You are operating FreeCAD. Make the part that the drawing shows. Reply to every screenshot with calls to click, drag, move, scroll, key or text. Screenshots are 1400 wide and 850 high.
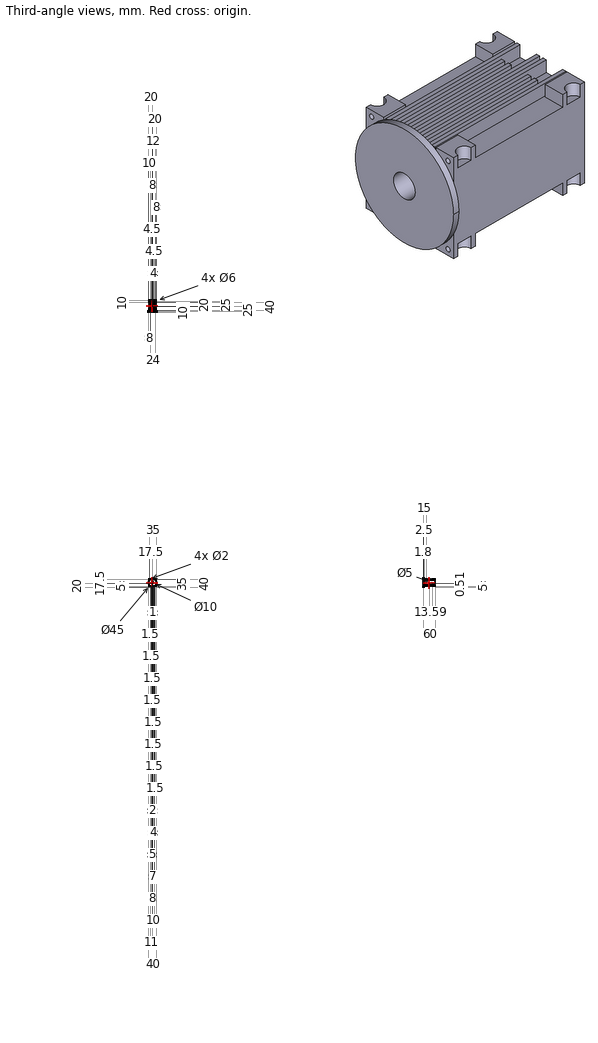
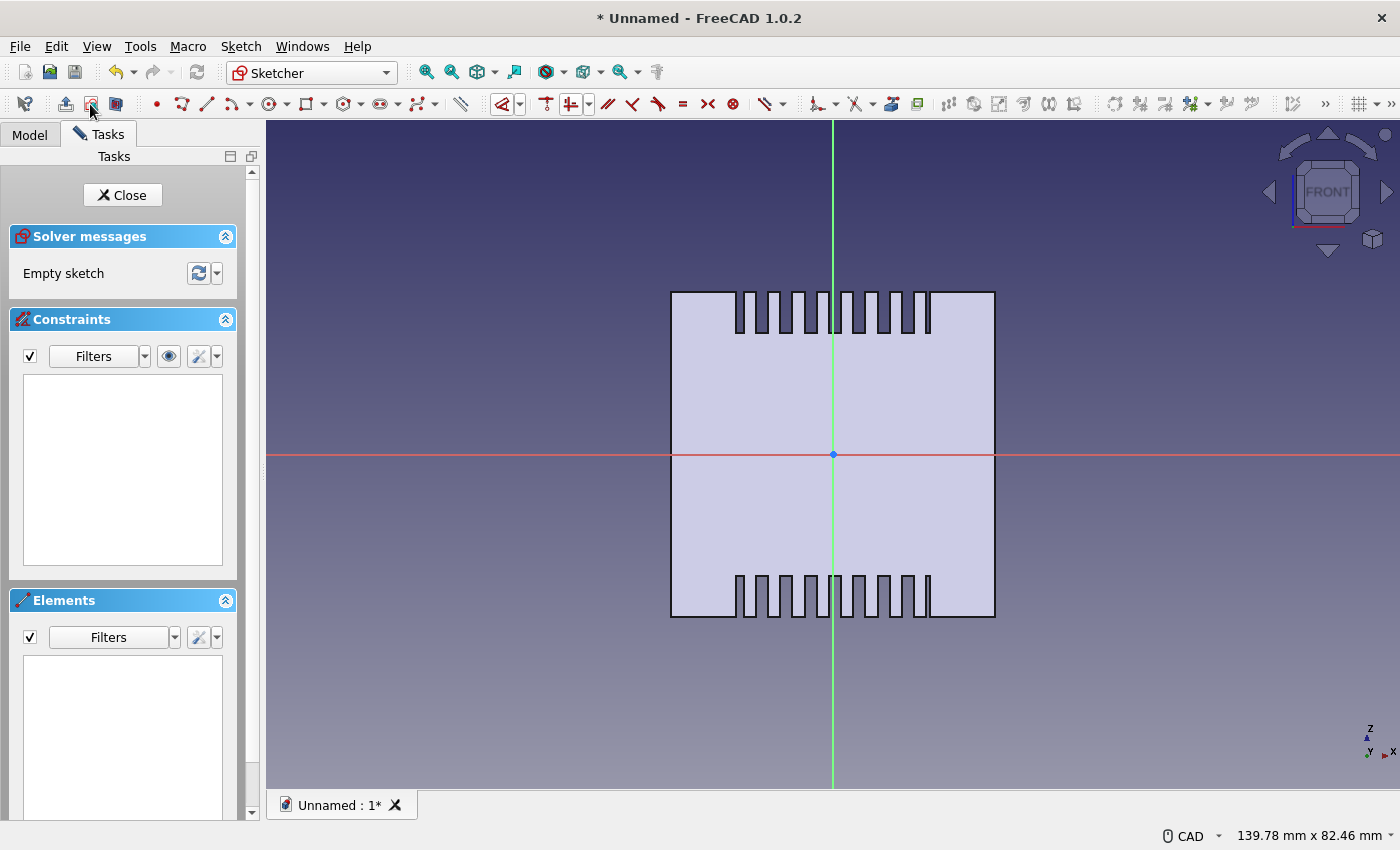
click(268, 104)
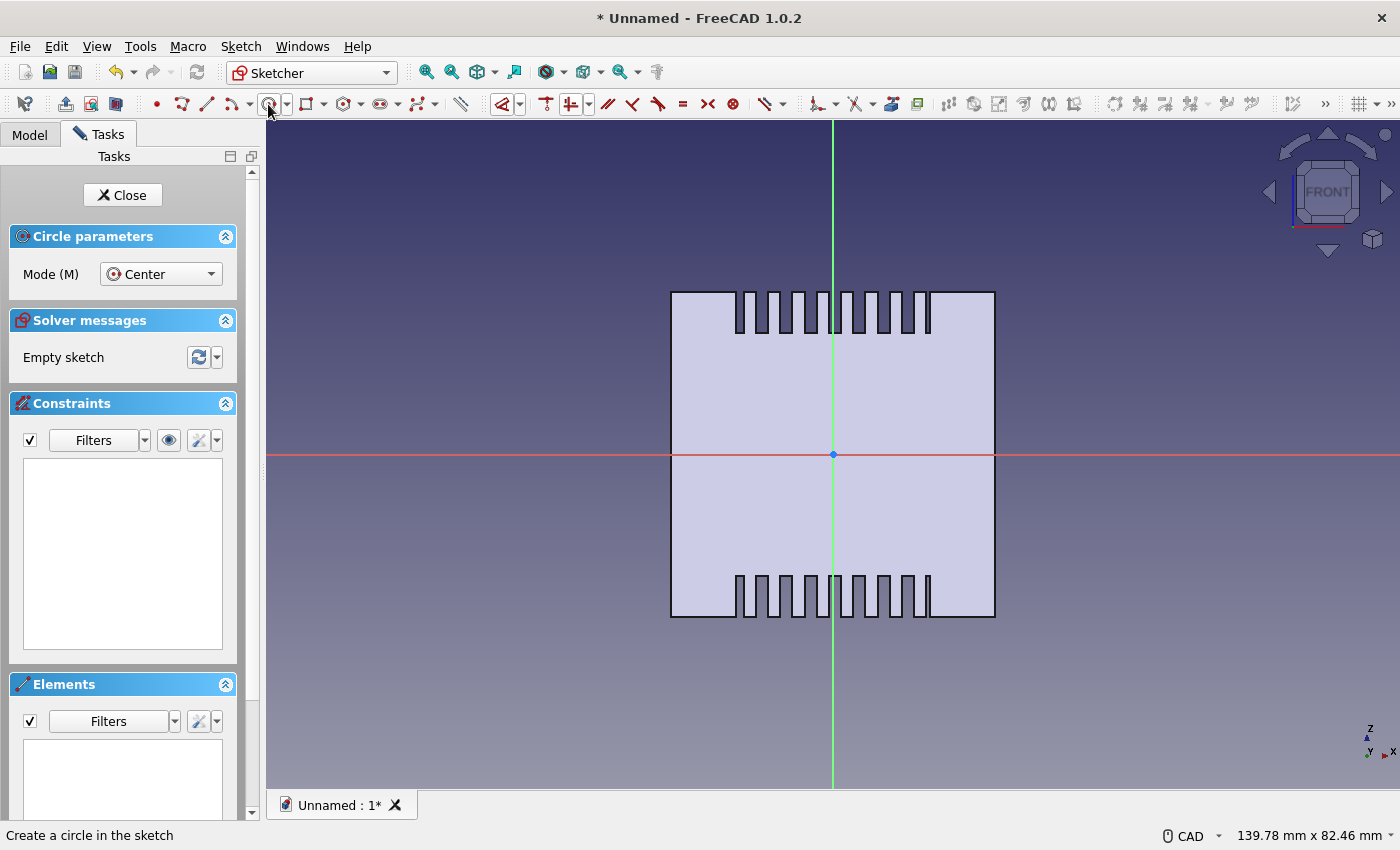
click(833, 454)
click(962, 325)
key(Escape)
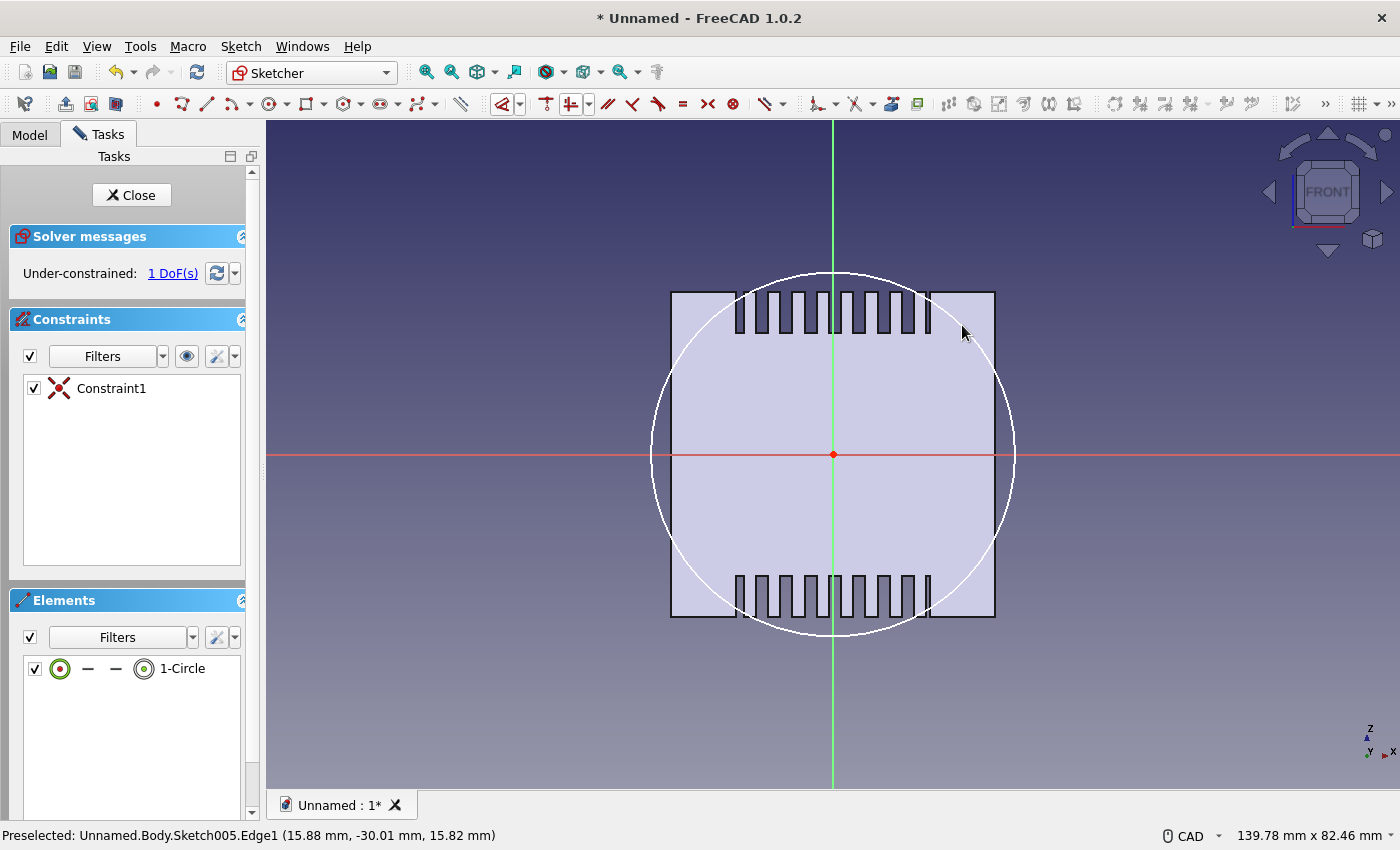
click(961, 325)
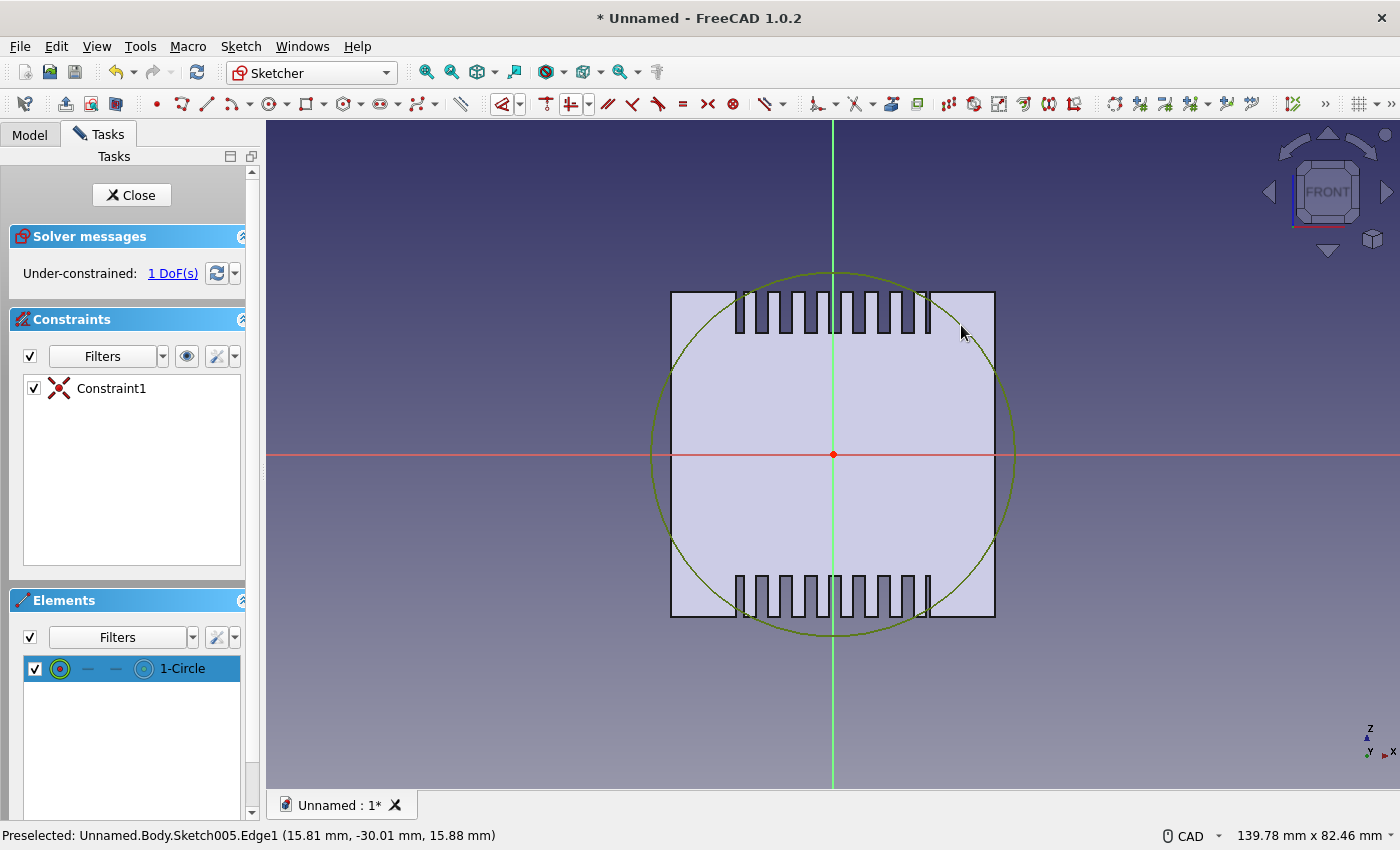
click(520, 104)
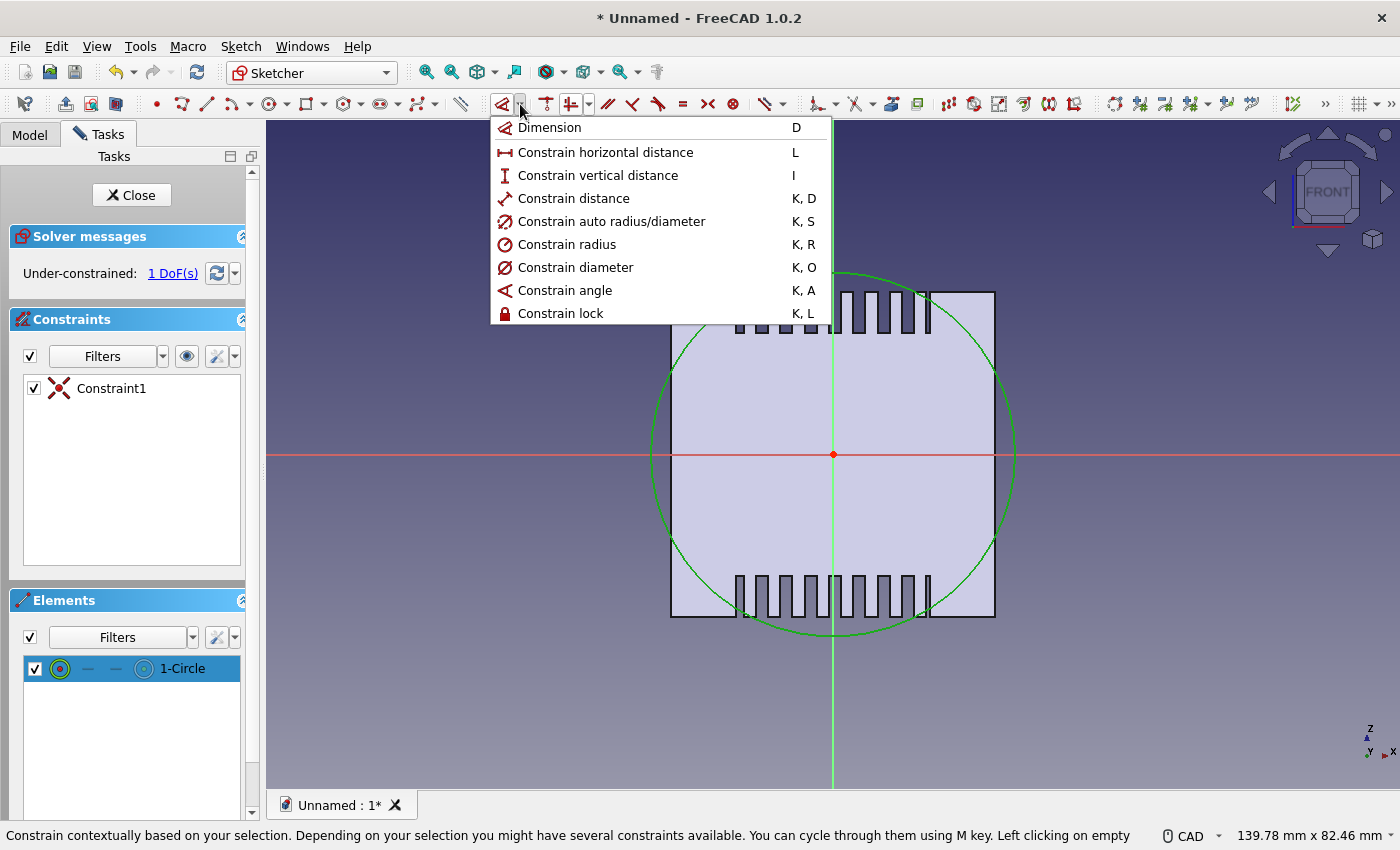
click(661, 268)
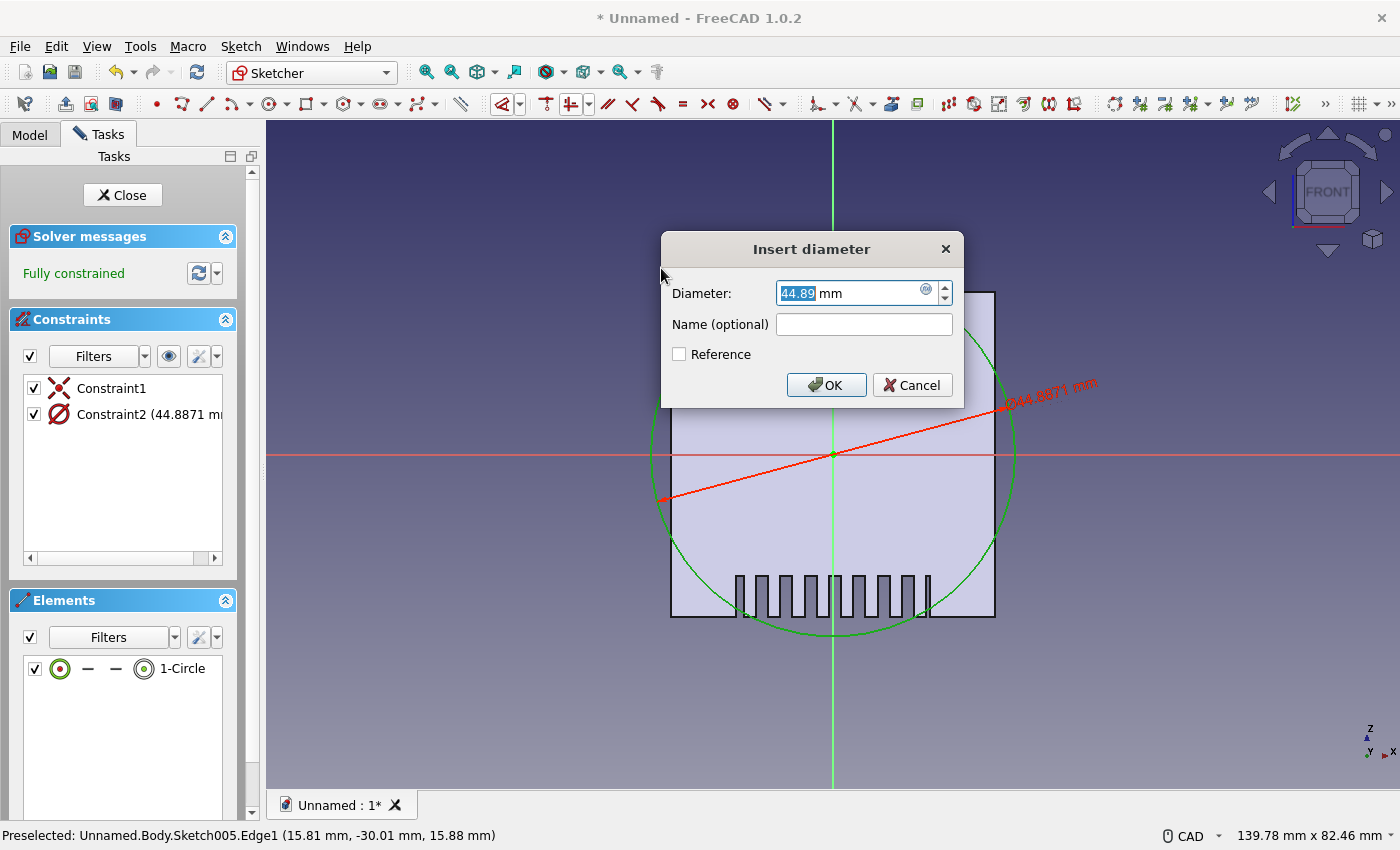
text(45)
key(Return)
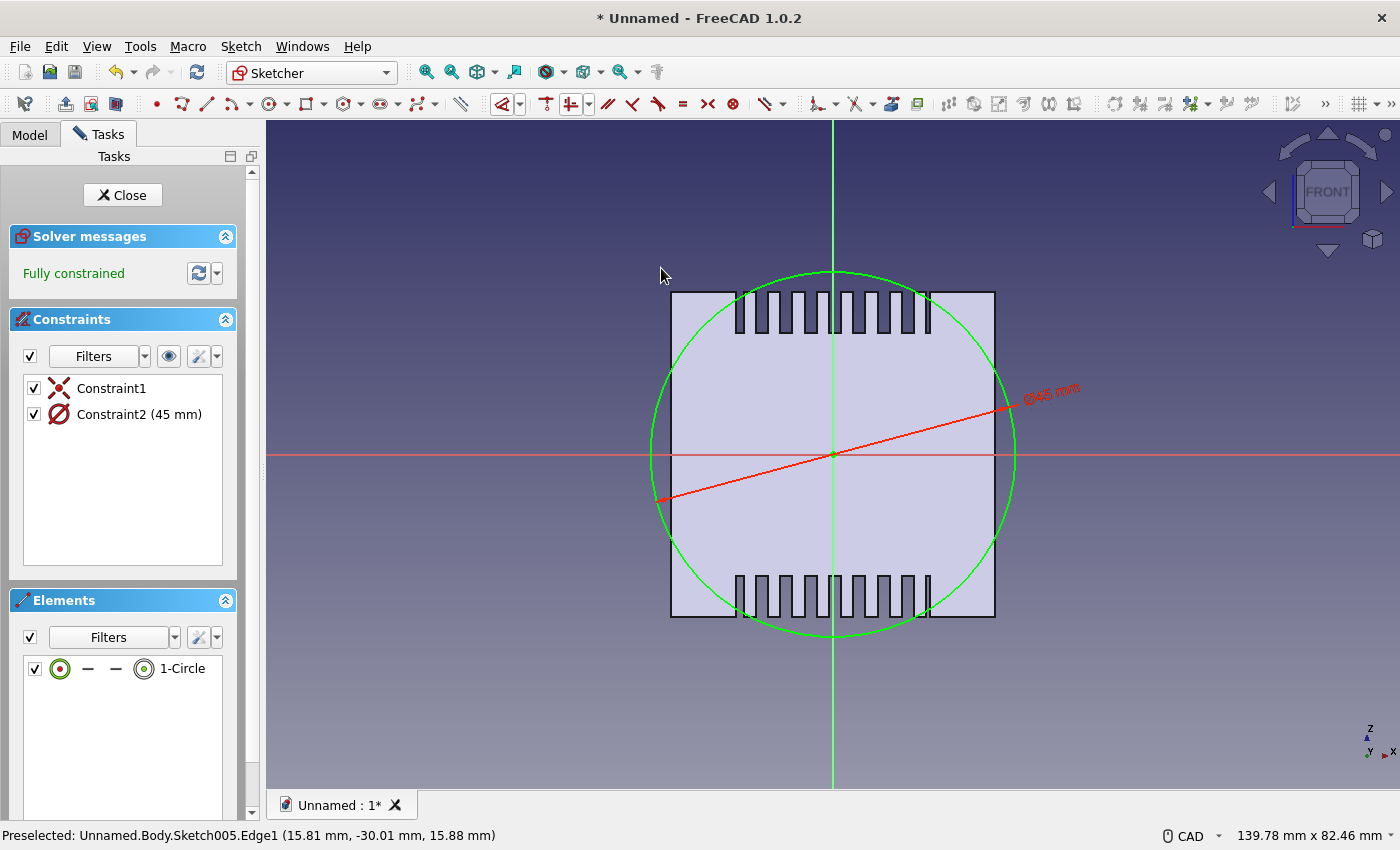
click(123, 195)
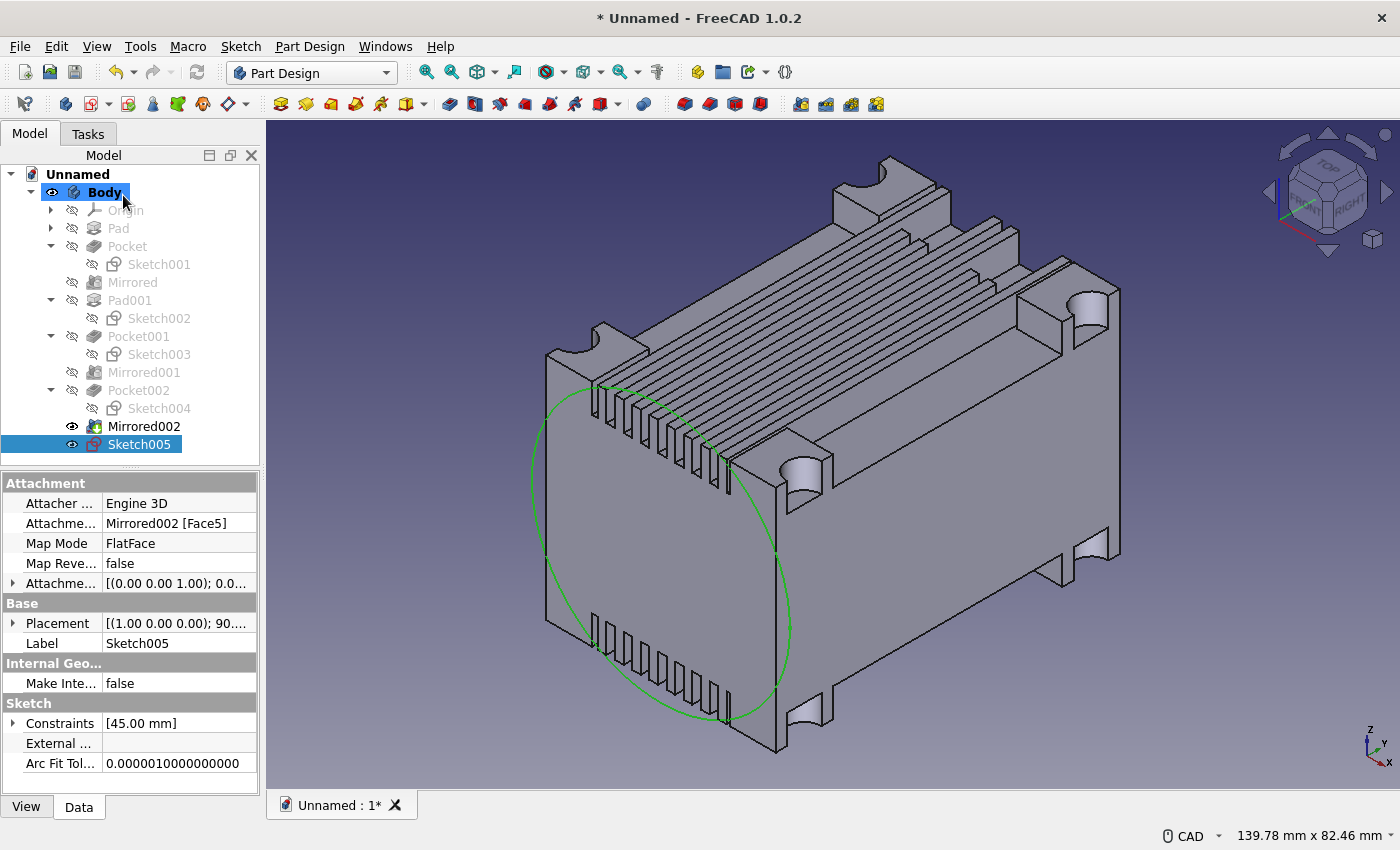
click(281, 104)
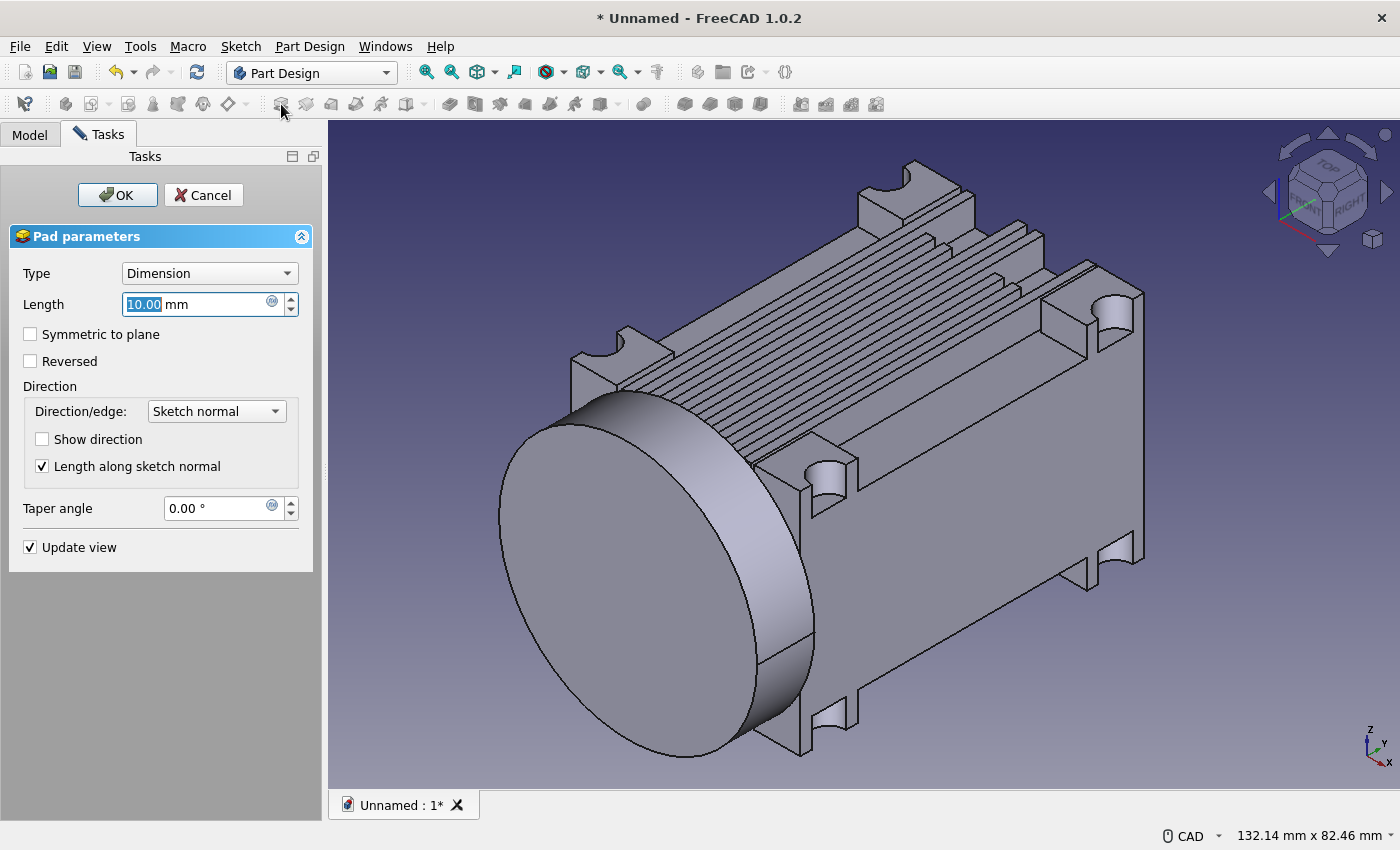
text(2.5)
key(Tab)